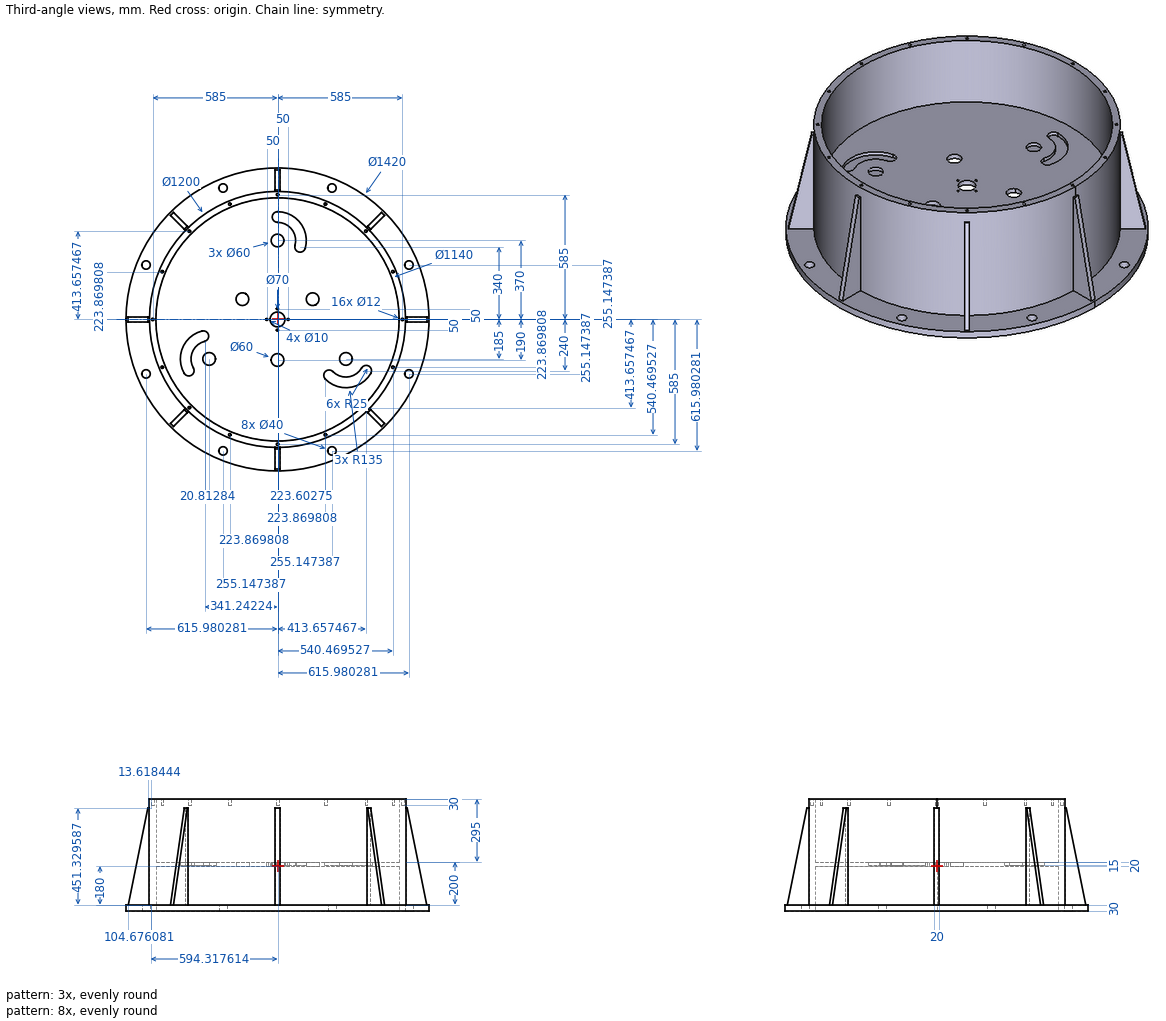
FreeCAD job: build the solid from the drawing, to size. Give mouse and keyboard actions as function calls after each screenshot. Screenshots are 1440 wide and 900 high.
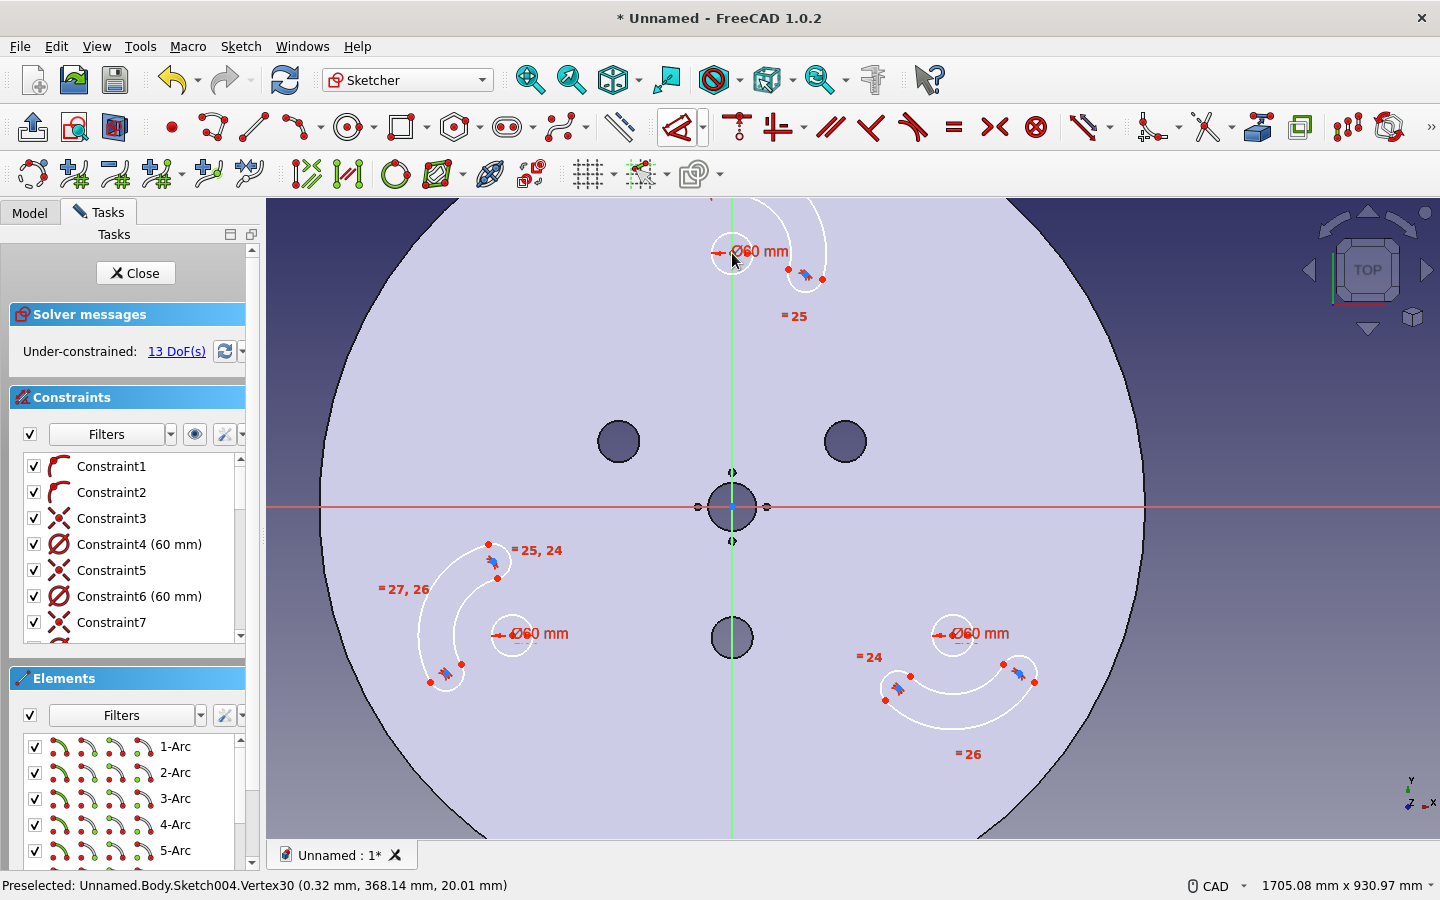
click(732, 769)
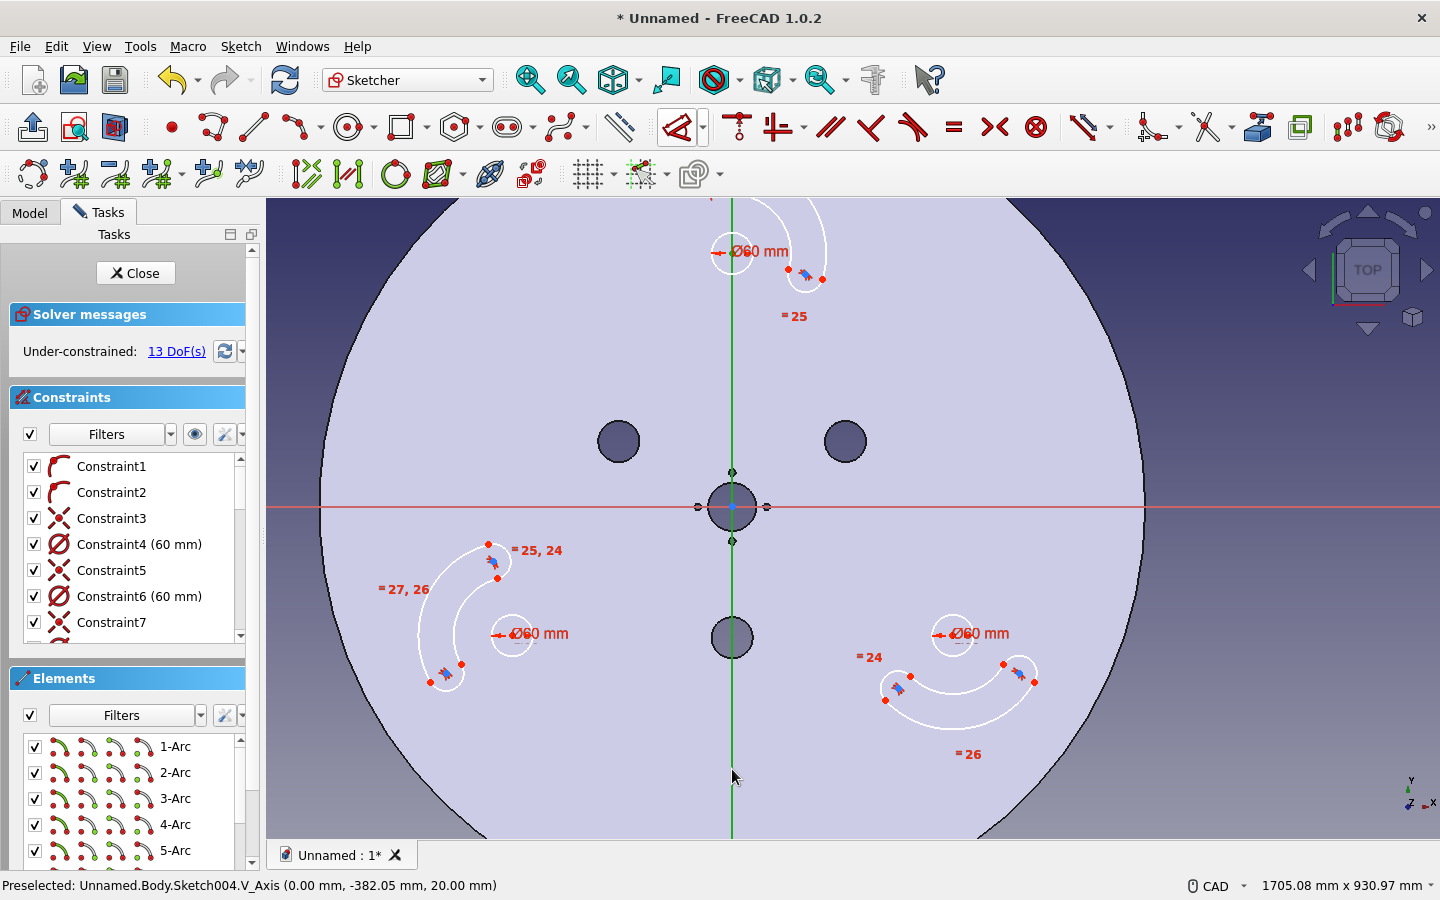
key(c)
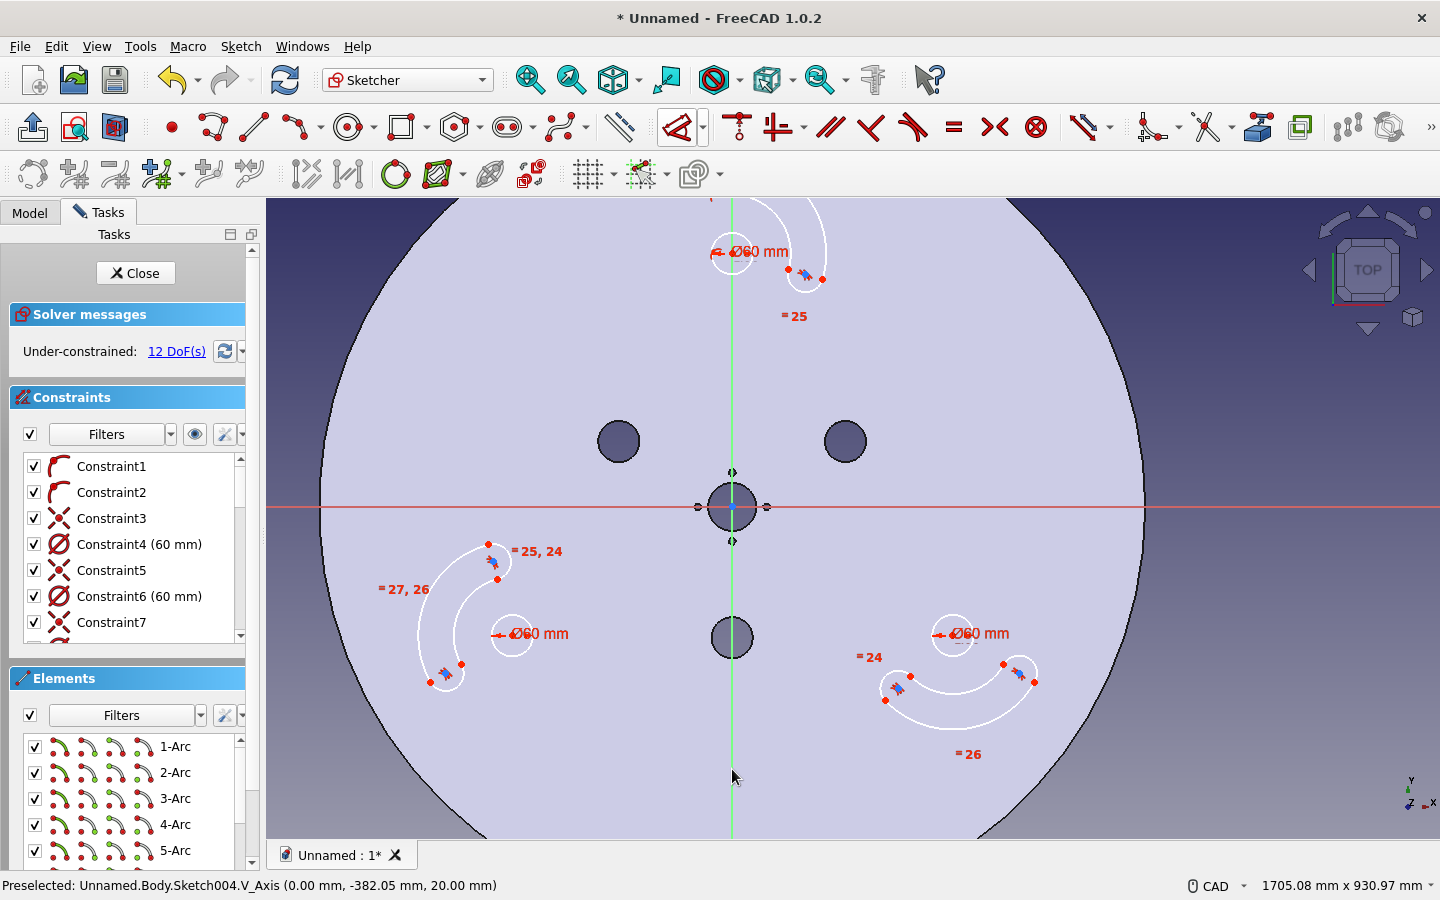
click(953, 636)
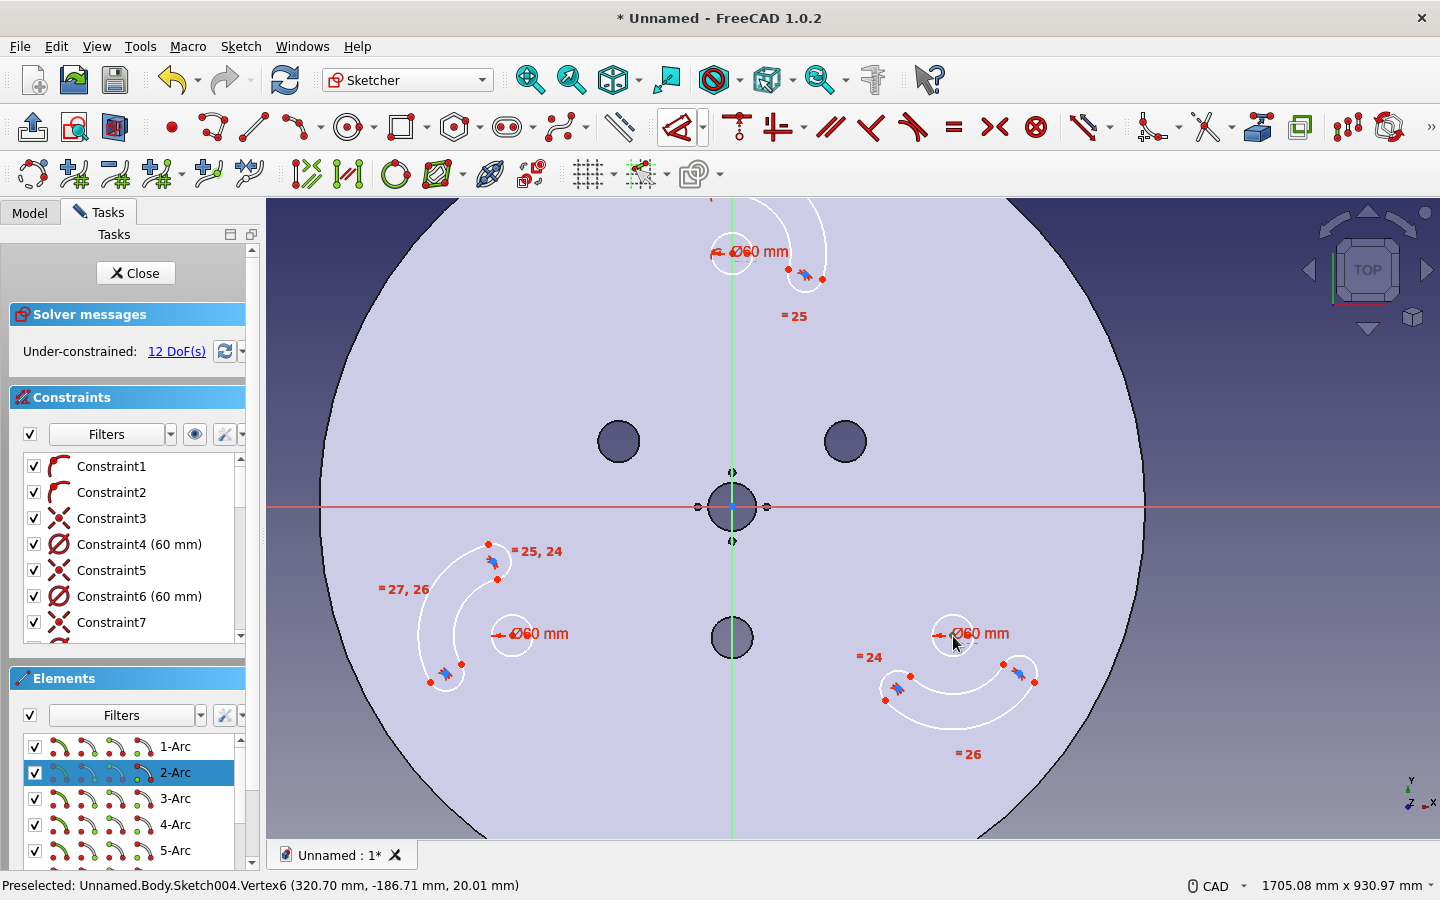
click(512, 636)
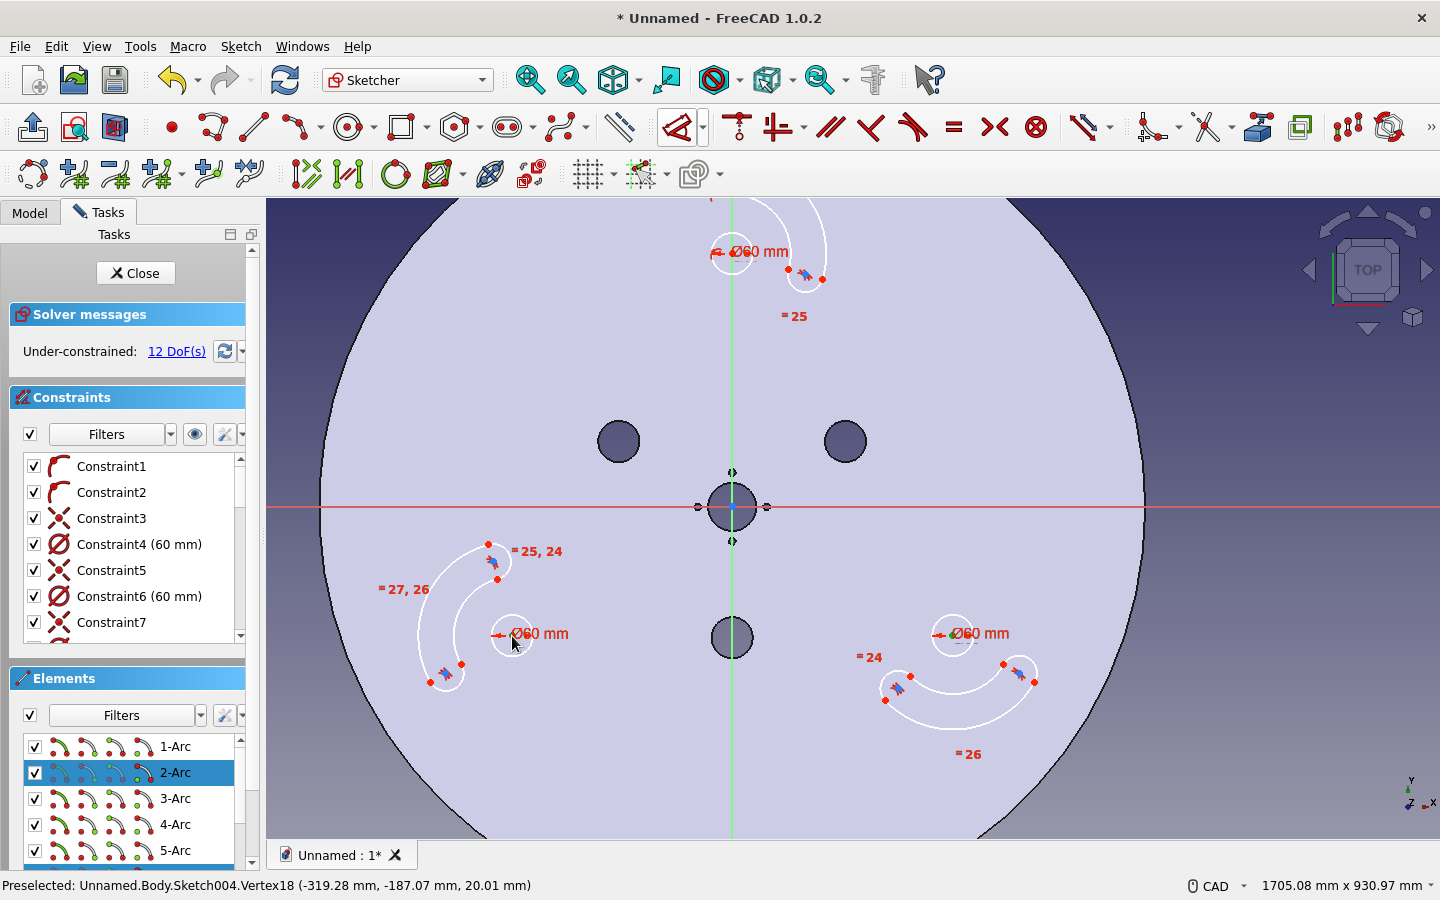
click(732, 769)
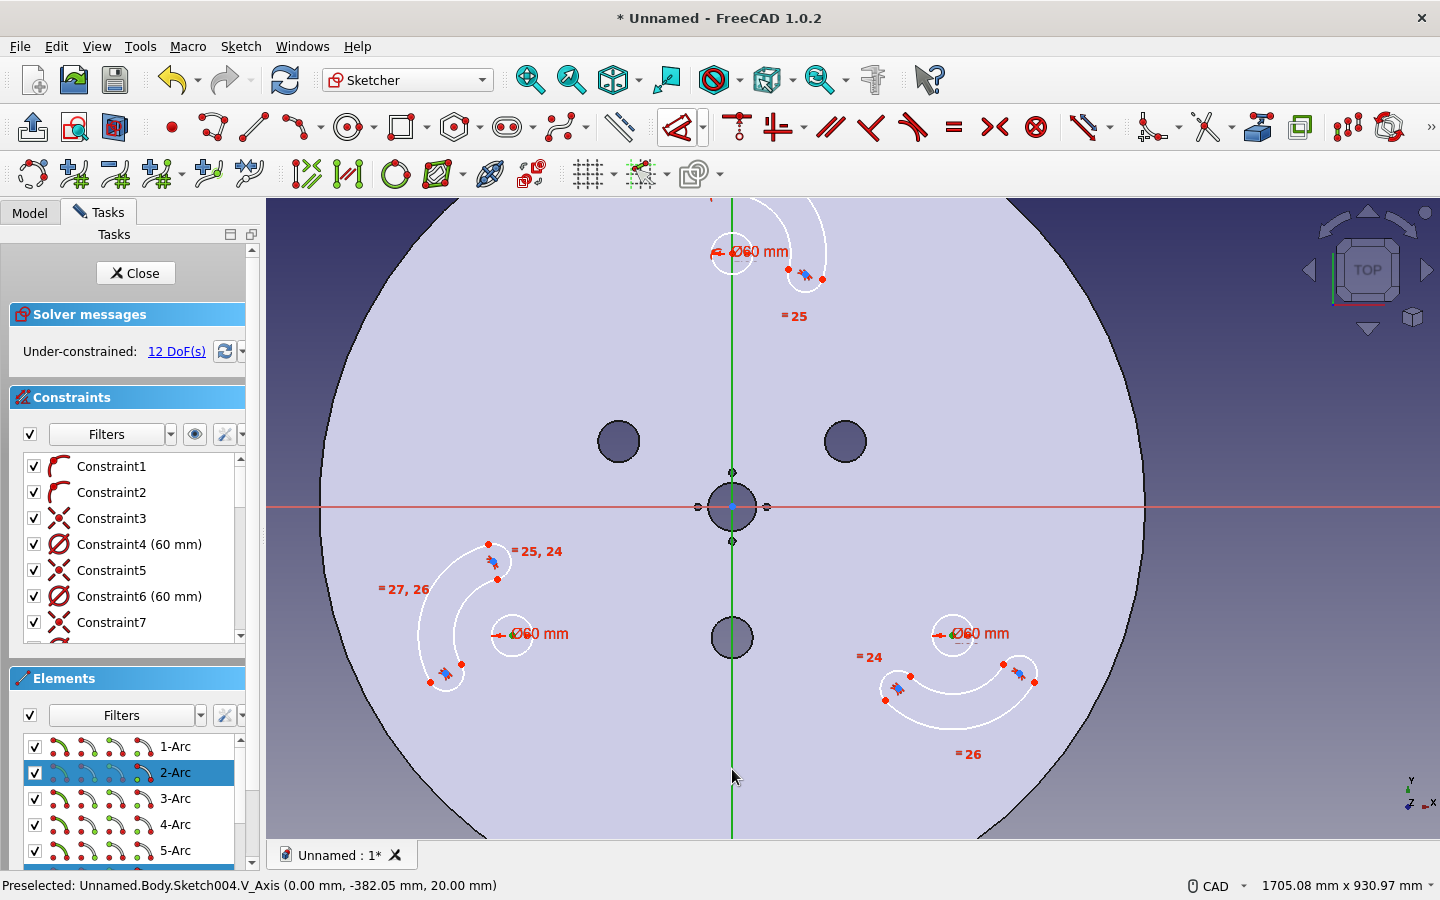
key(s)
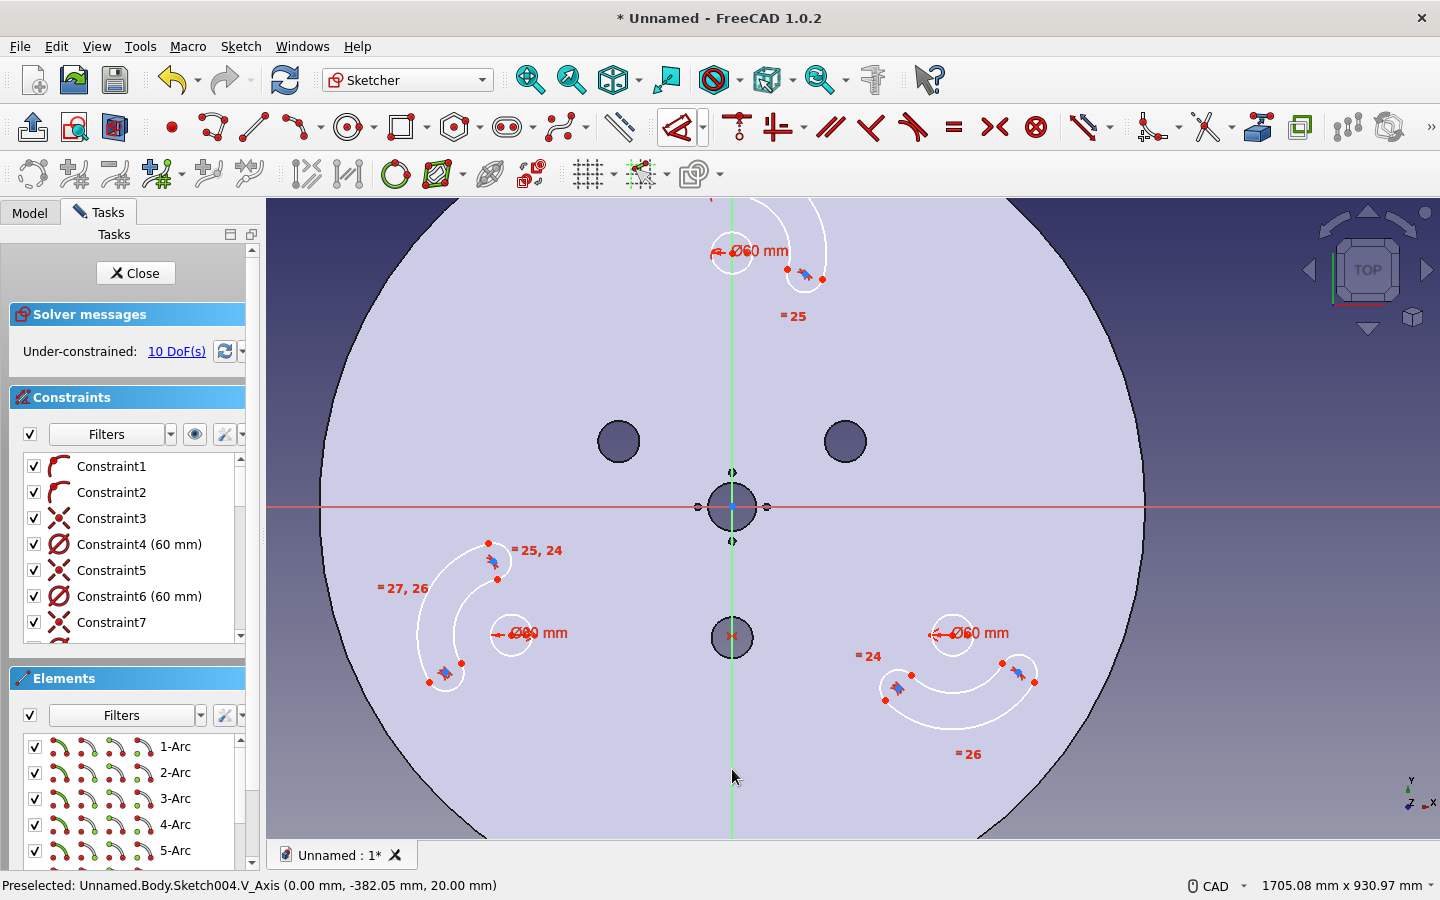
scroll(896, 670, up, 5)